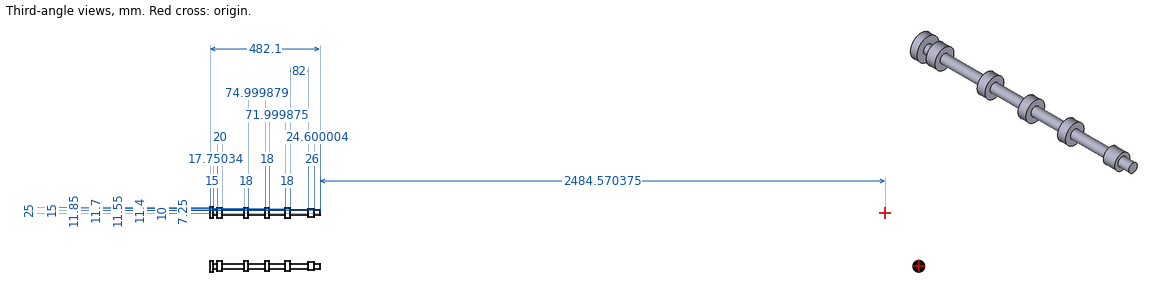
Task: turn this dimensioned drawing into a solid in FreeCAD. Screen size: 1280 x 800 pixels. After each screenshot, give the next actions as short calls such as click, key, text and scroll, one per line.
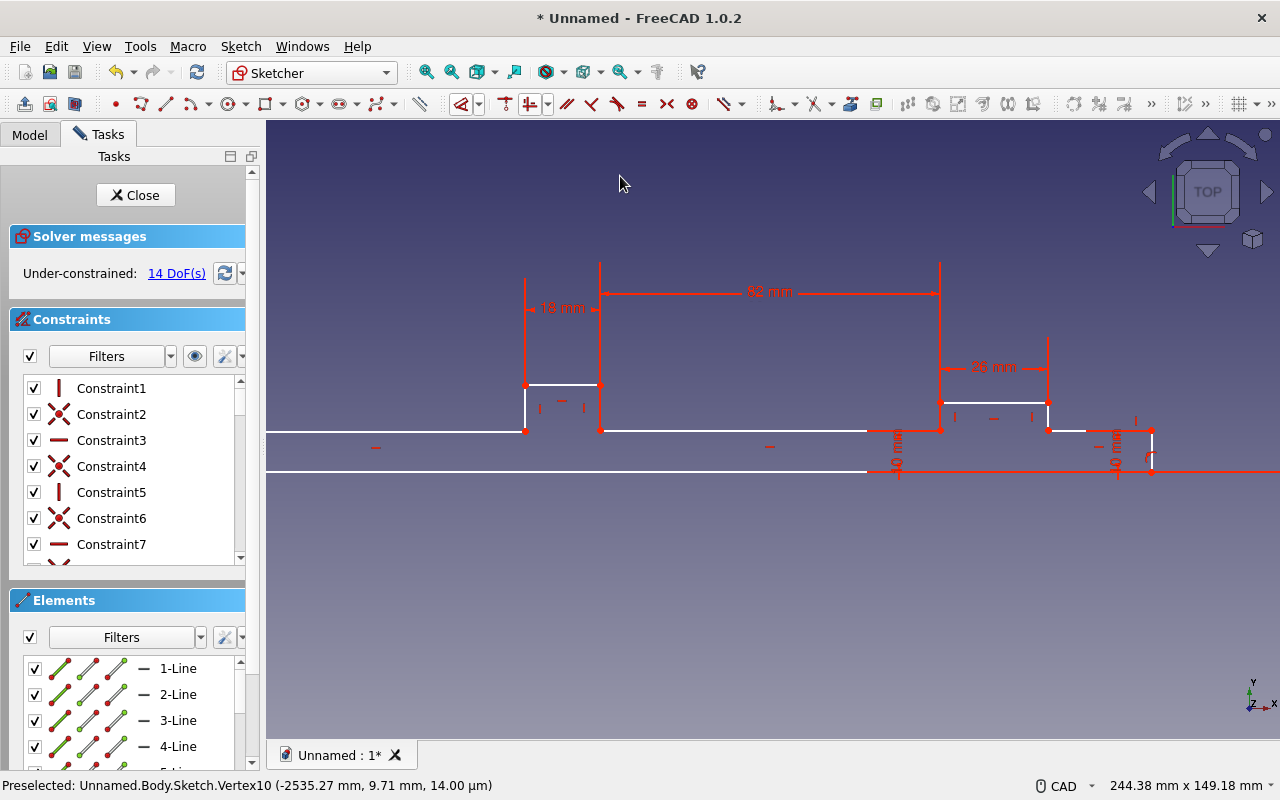
click(525, 432)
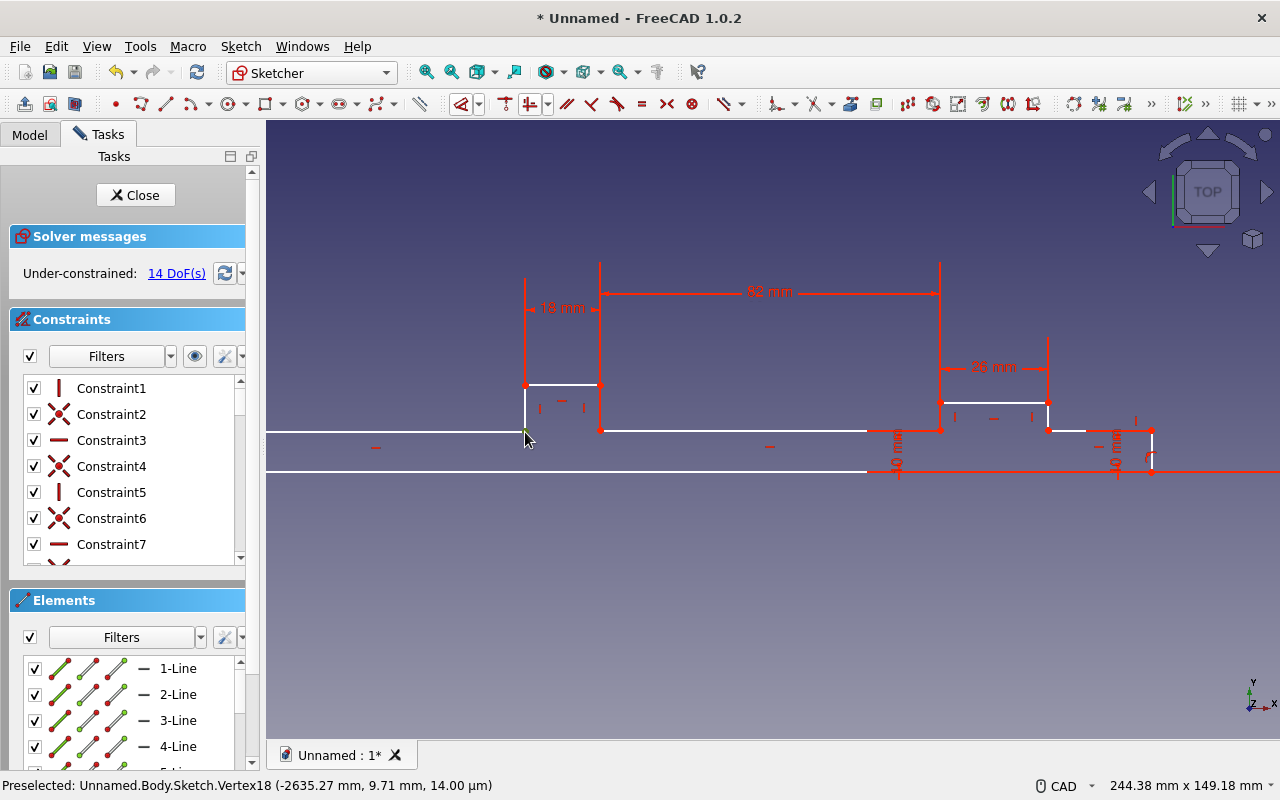
key(i)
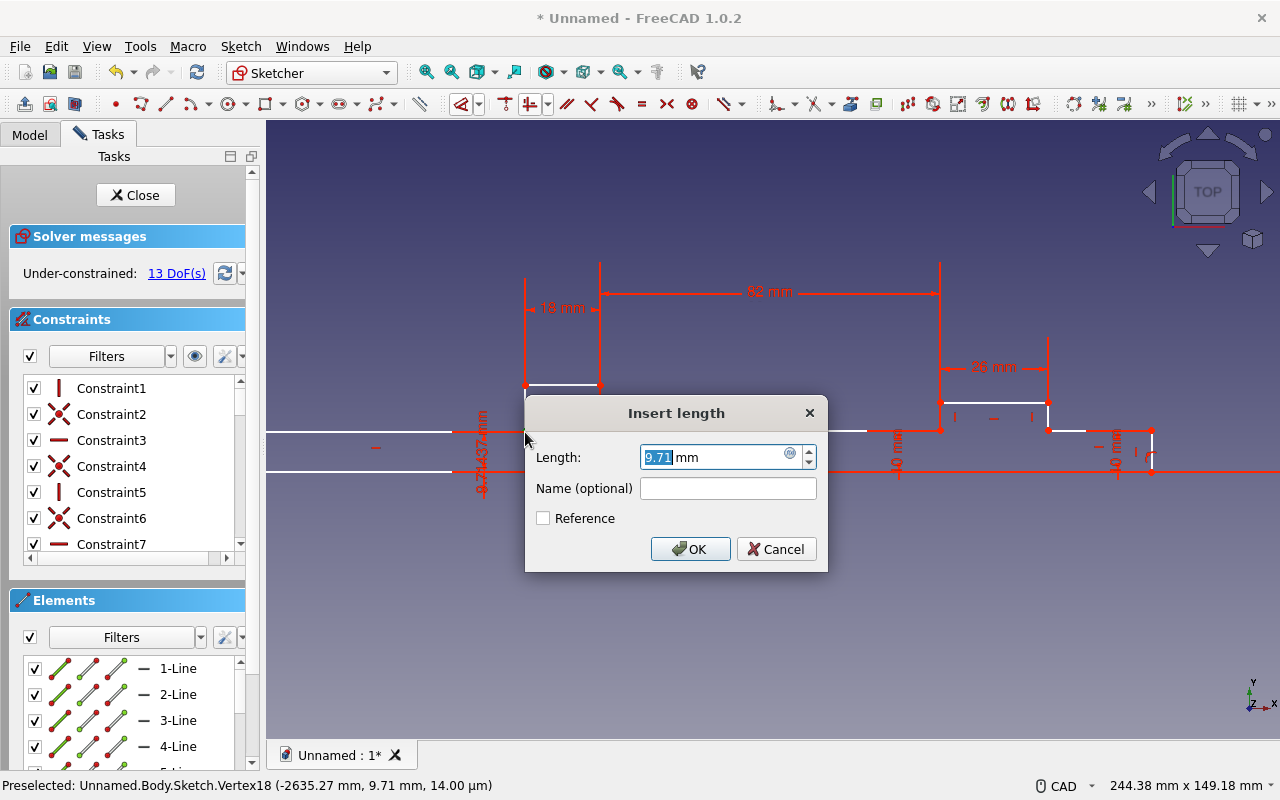
text(10)
key(Return)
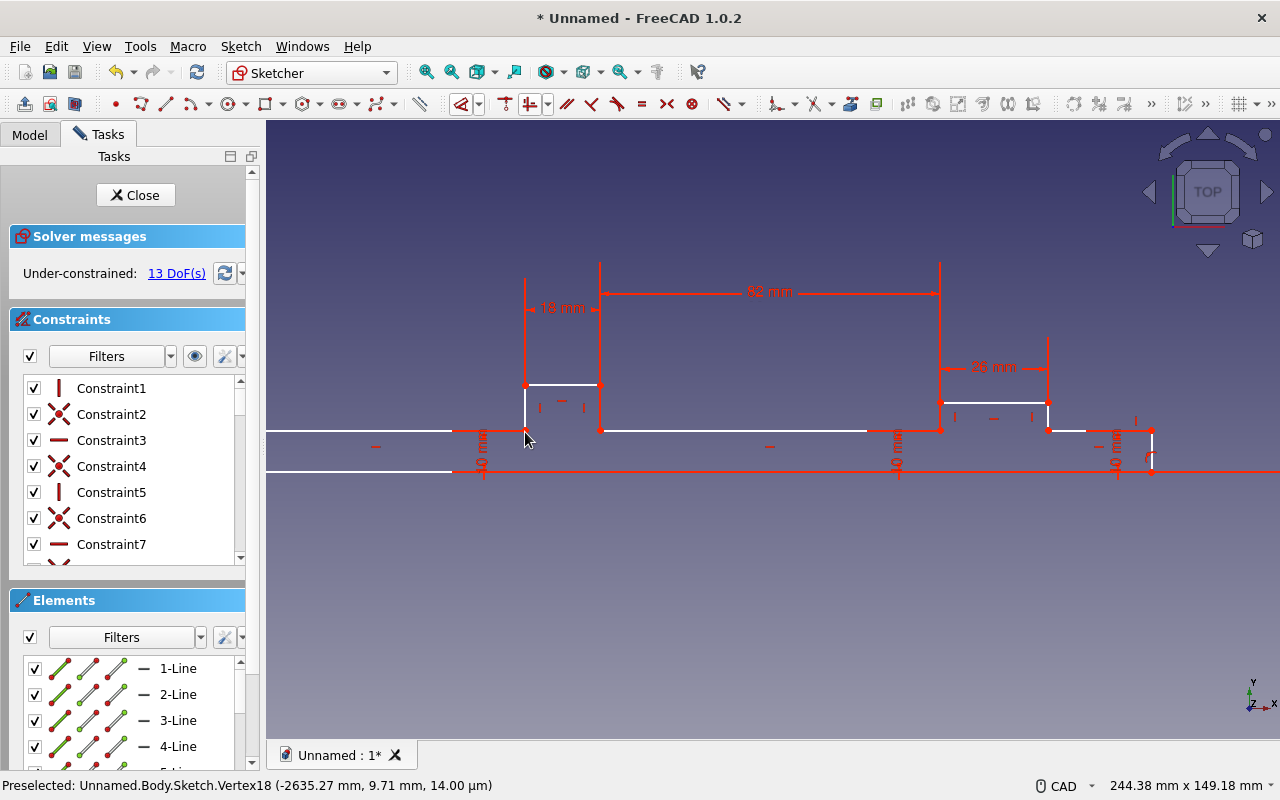
scroll(943, 433, down, 6)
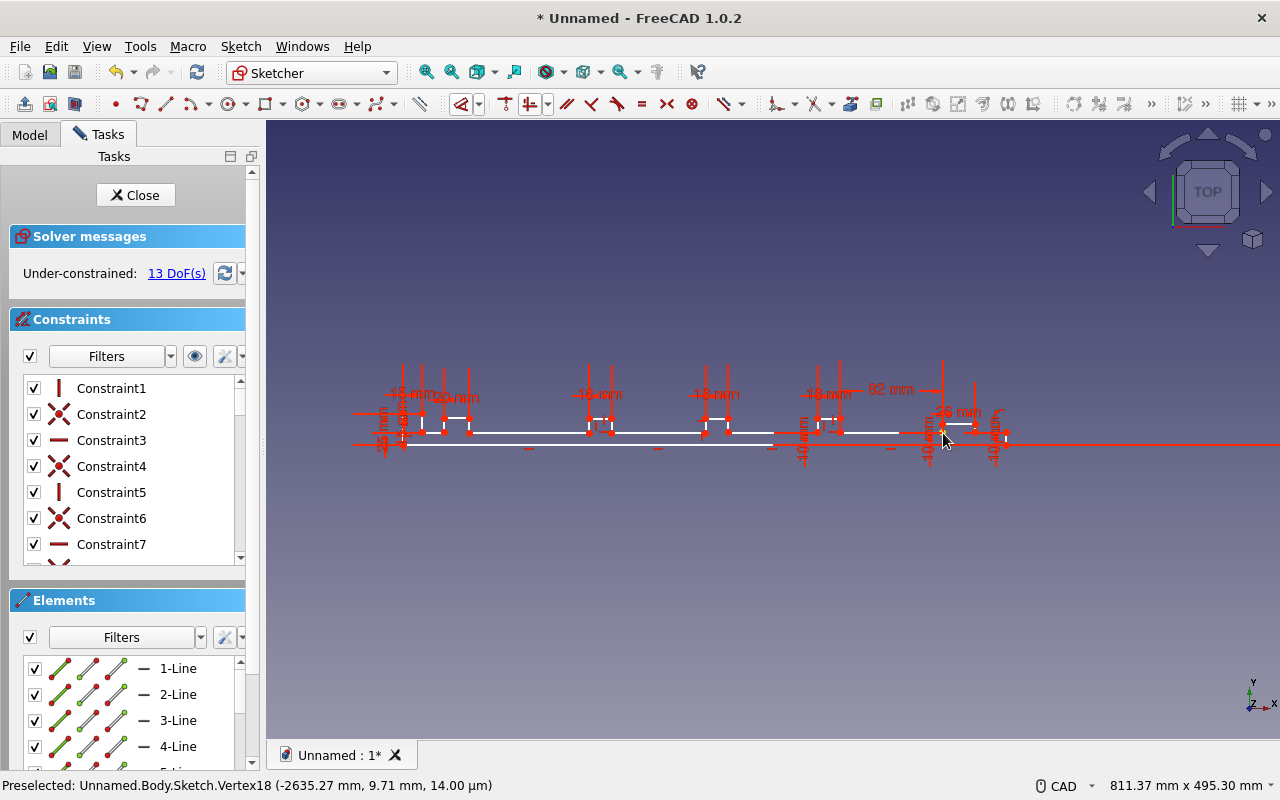
scroll(706, 433, up, 6)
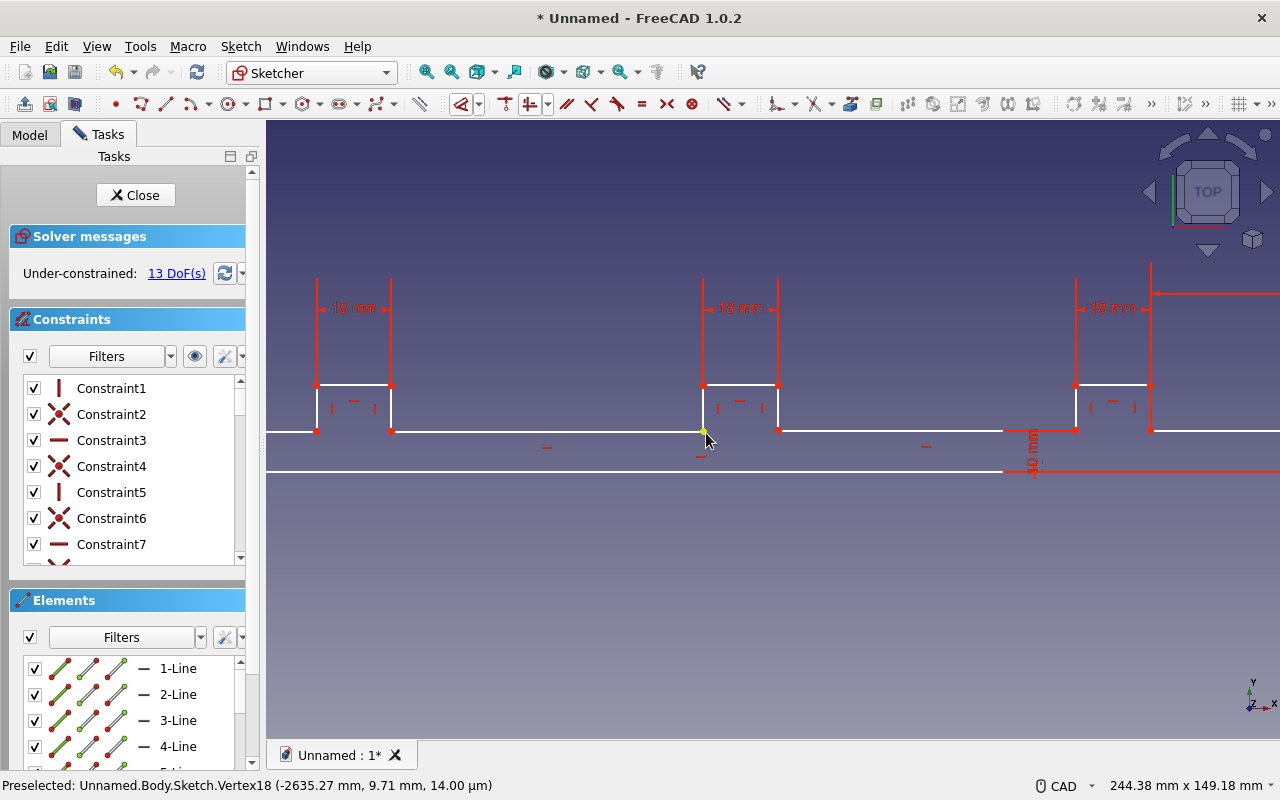
click(703, 432)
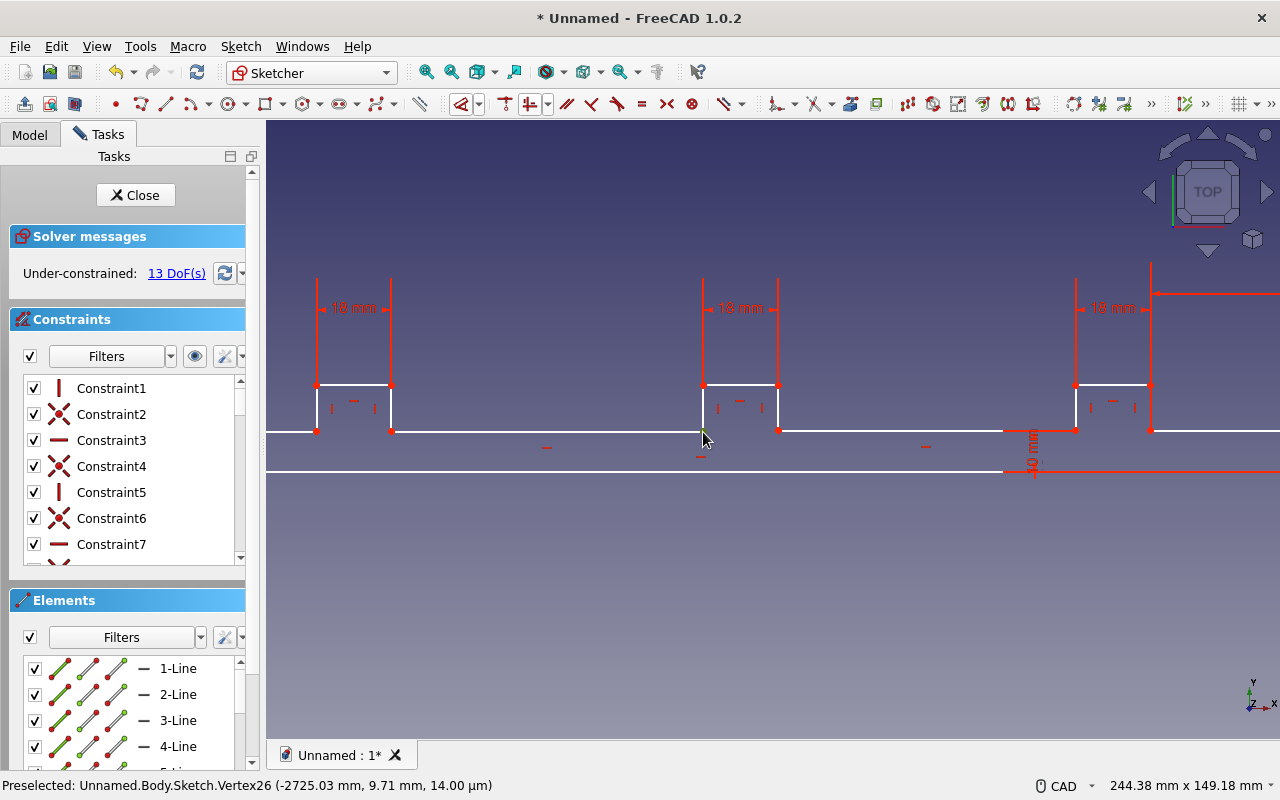
key(i)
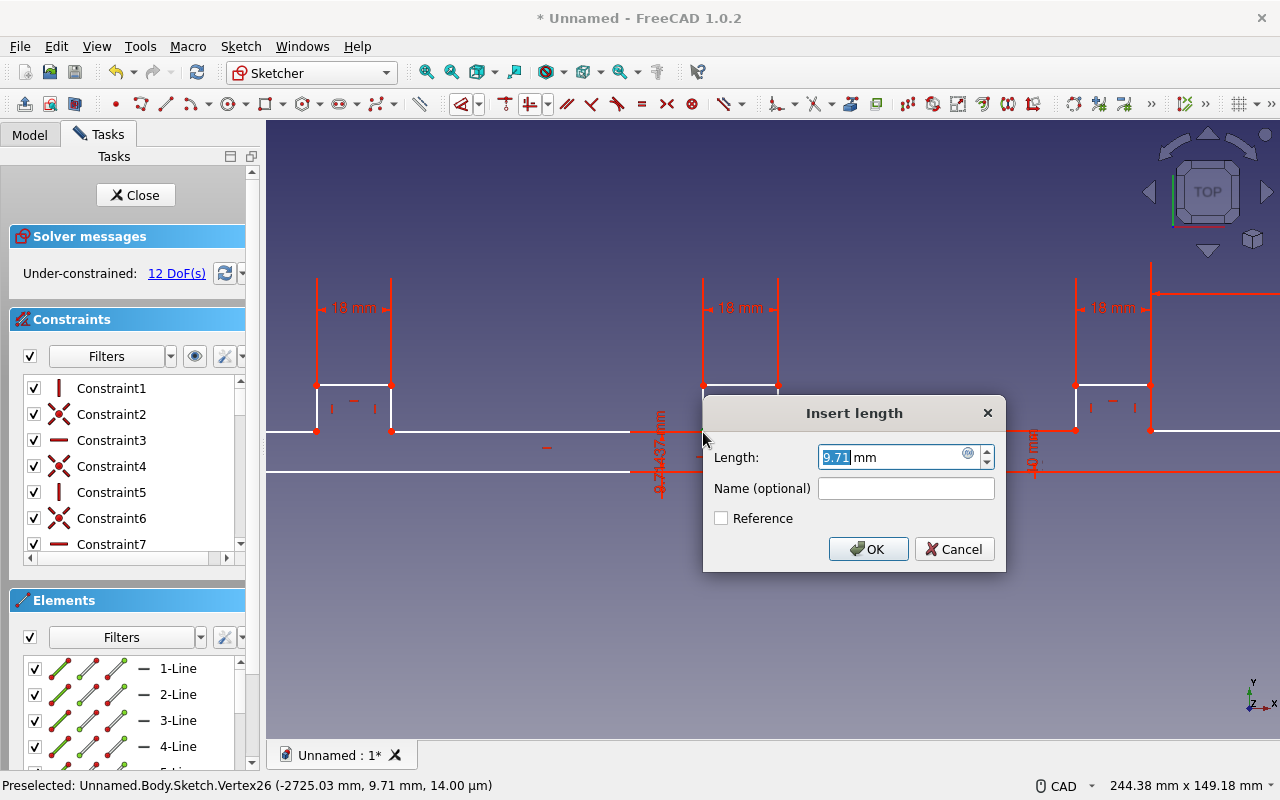
text(10)
key(Return)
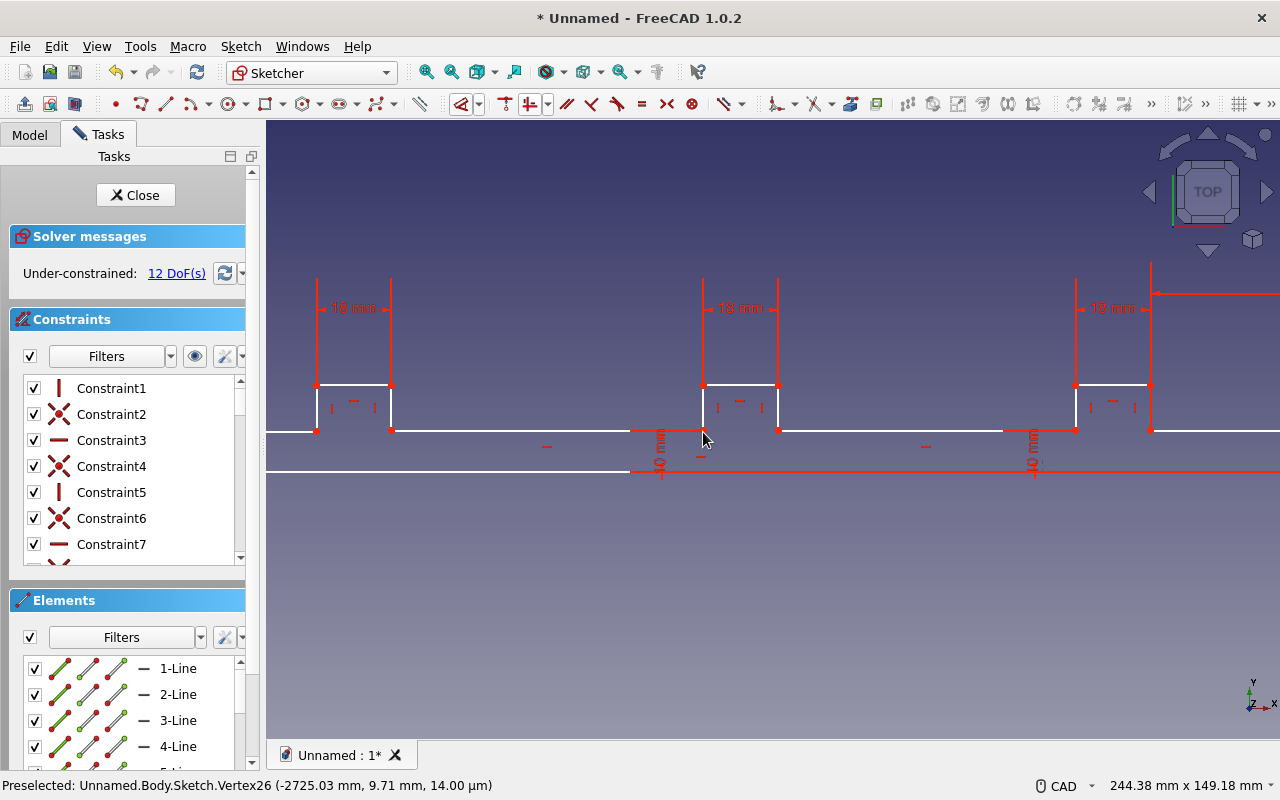
click(317, 432)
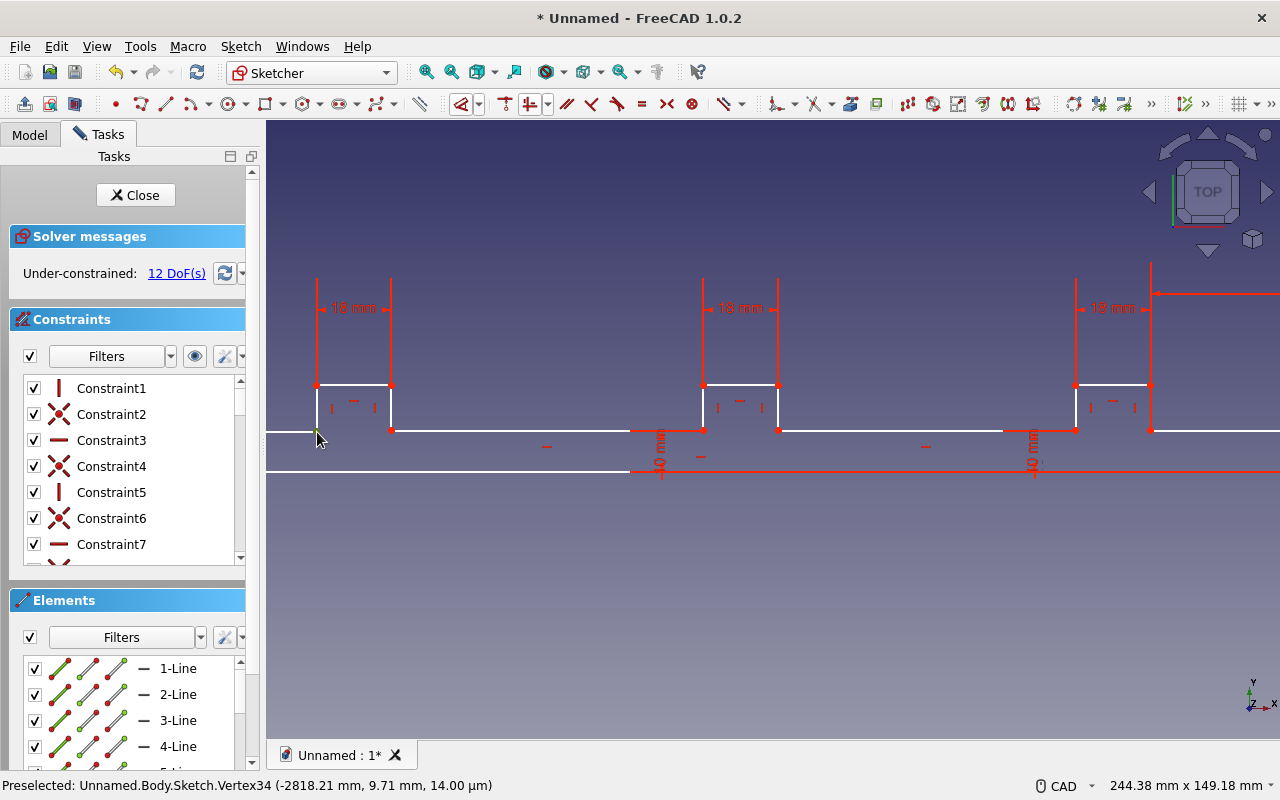
click(478, 104)